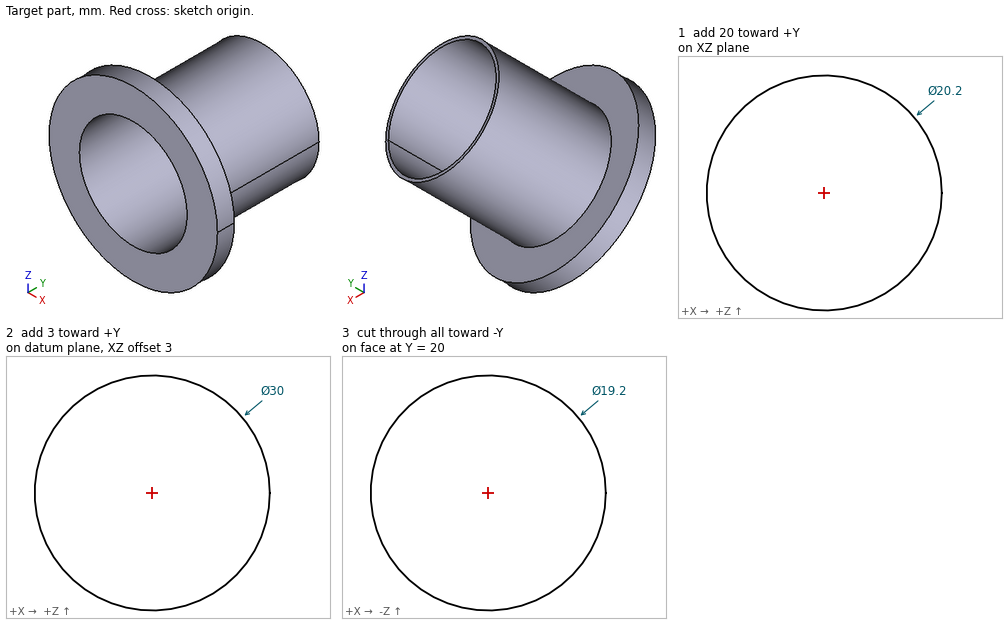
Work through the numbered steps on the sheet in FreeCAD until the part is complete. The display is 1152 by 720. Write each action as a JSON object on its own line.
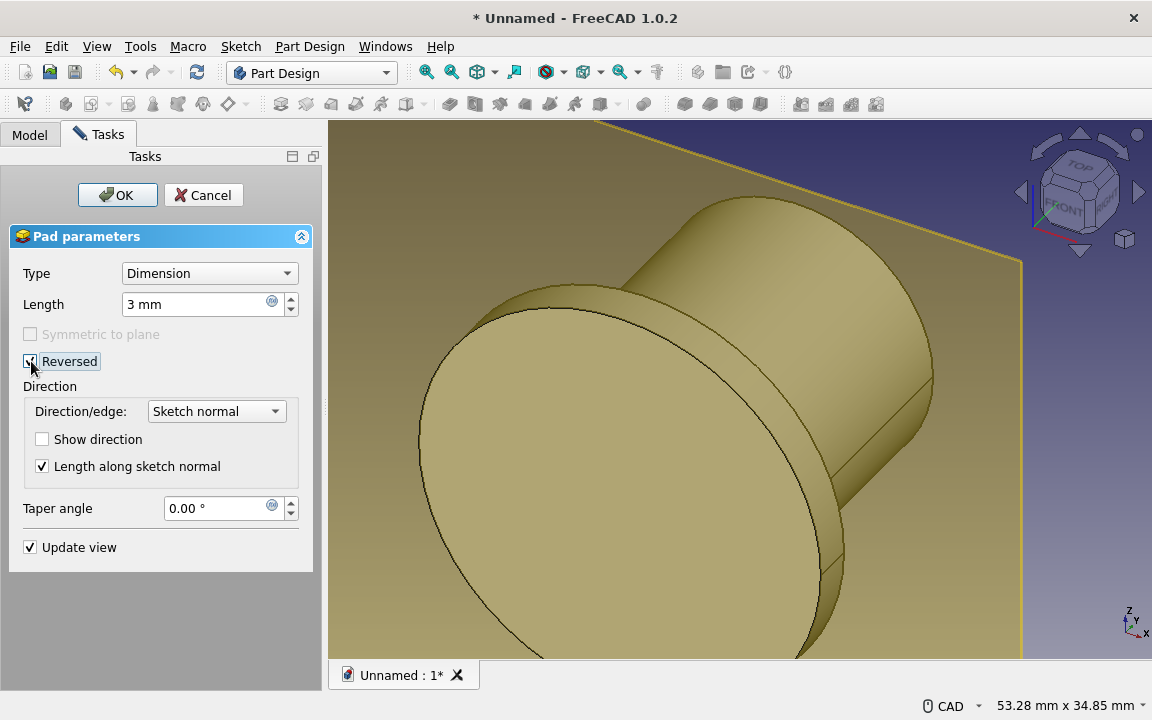
{"action": "left_click", "coordinate": [118, 195]}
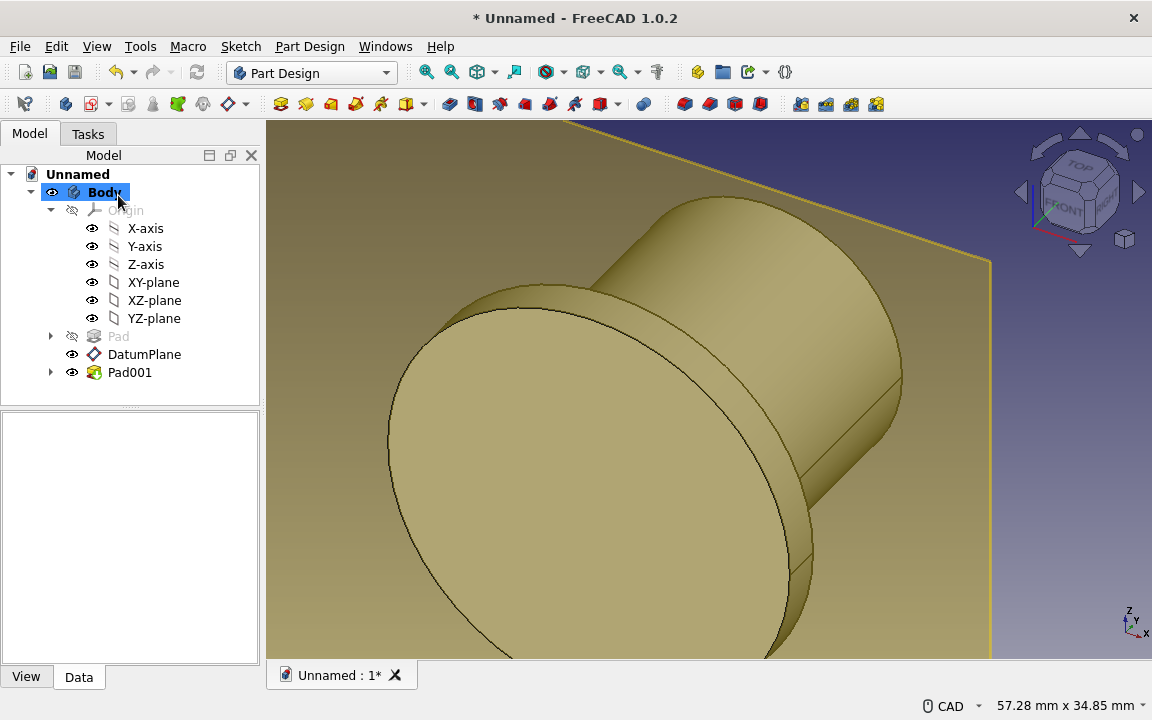
{"action": "left_click", "coordinate": [117, 354]}
{"action": "key", "text": "space"}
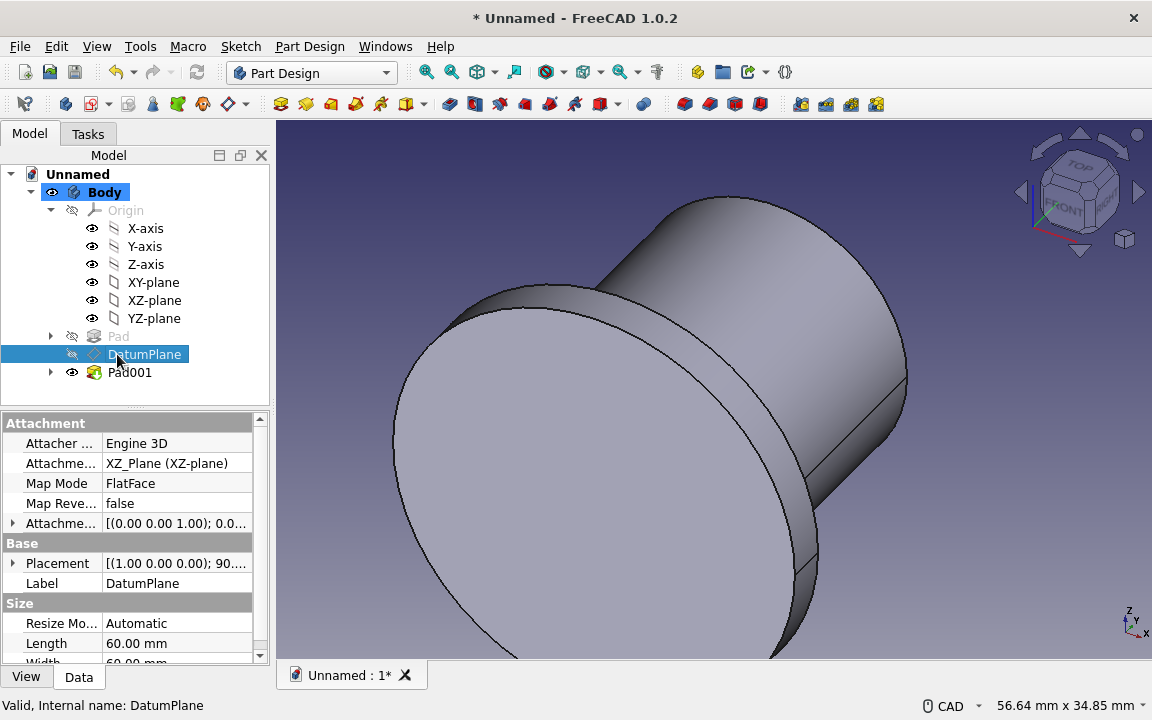
{"action": "key", "text": "v f"}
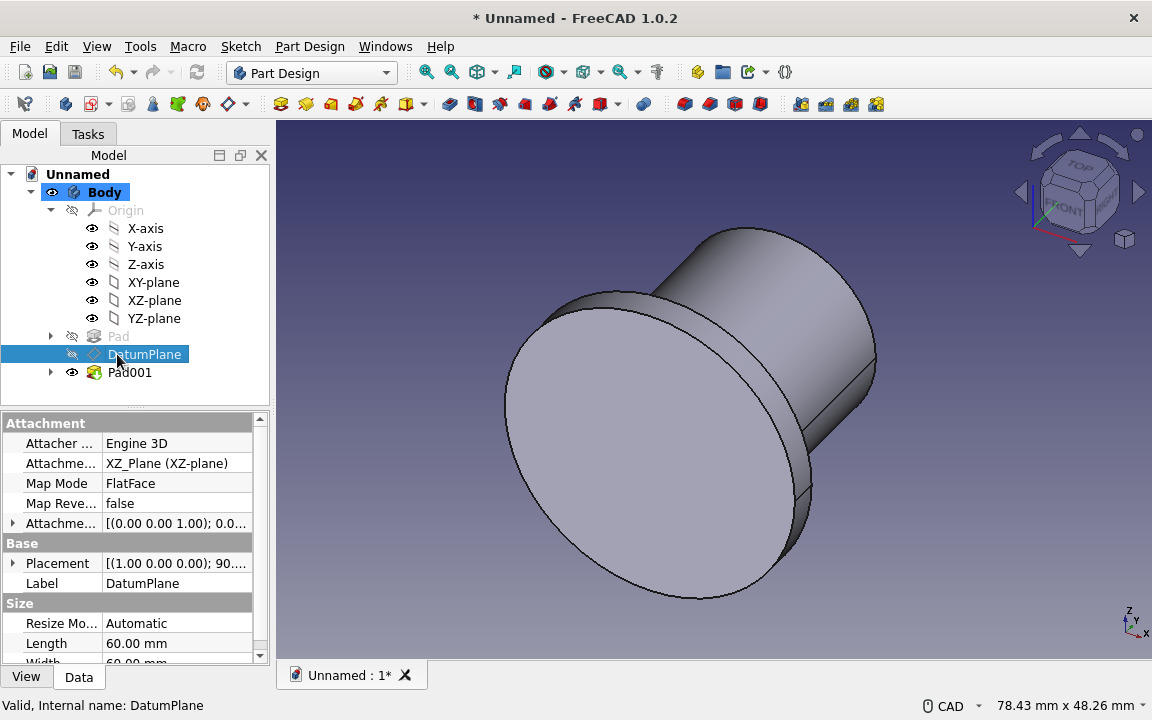
{"action": "key", "text": "4"}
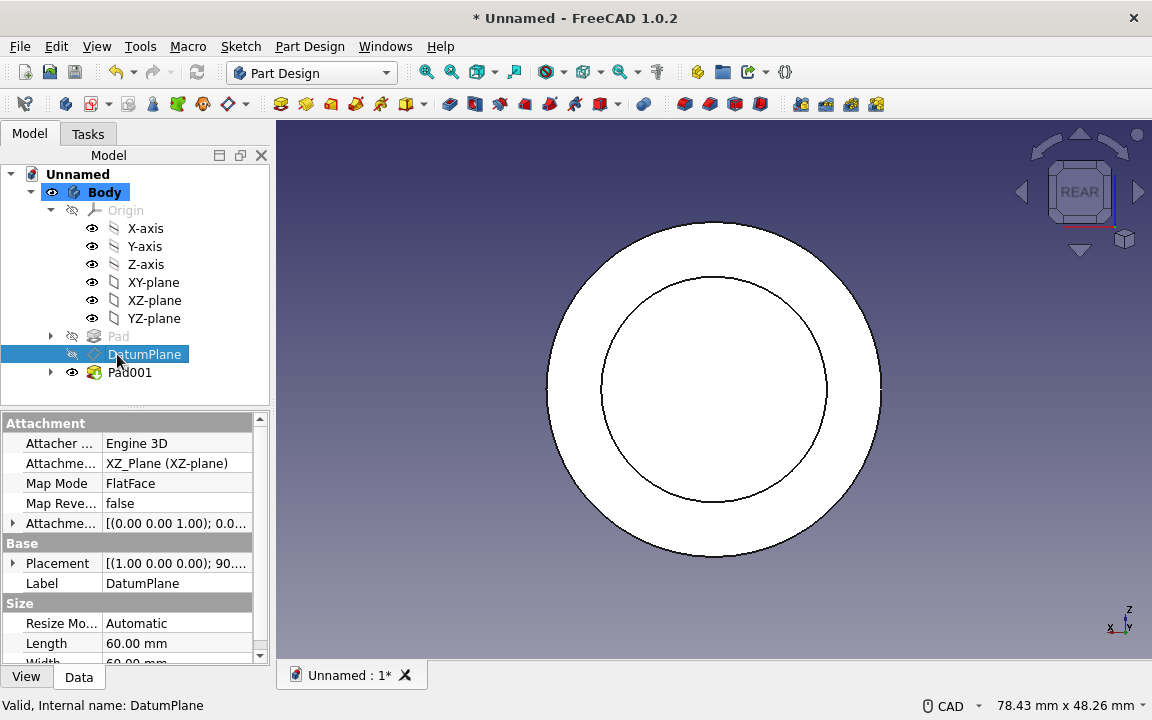
{"action": "left_click", "coordinate": [714, 389]}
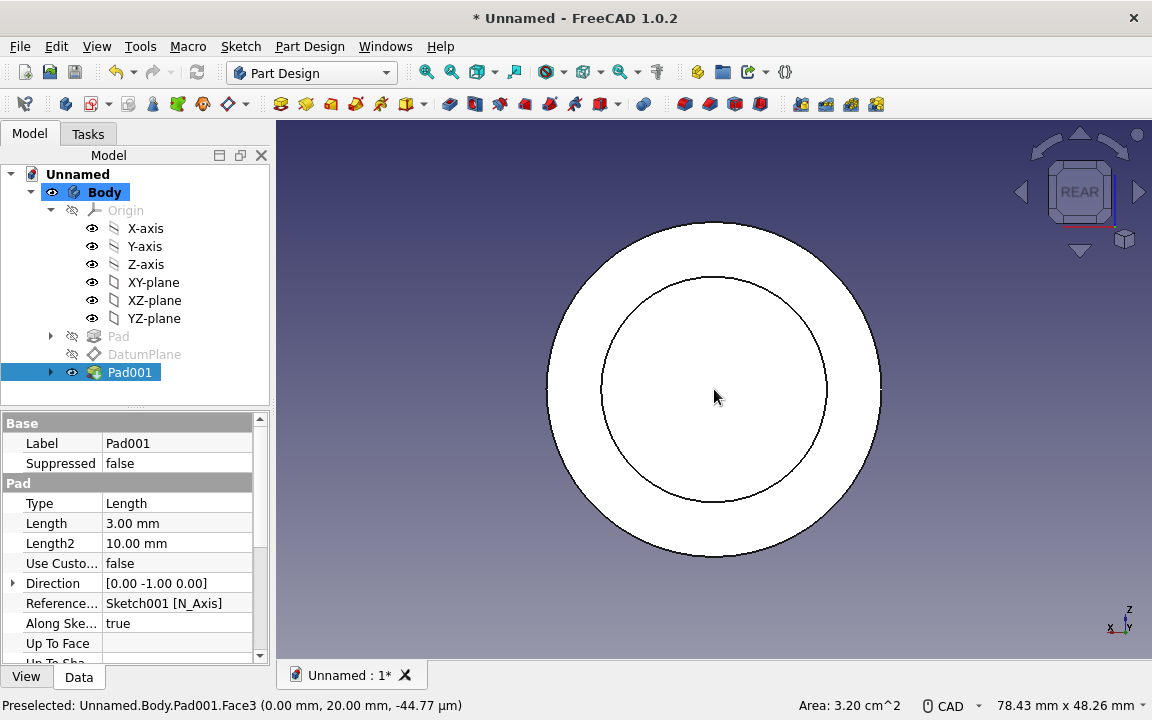
{"action": "left_click", "coordinate": [90, 104]}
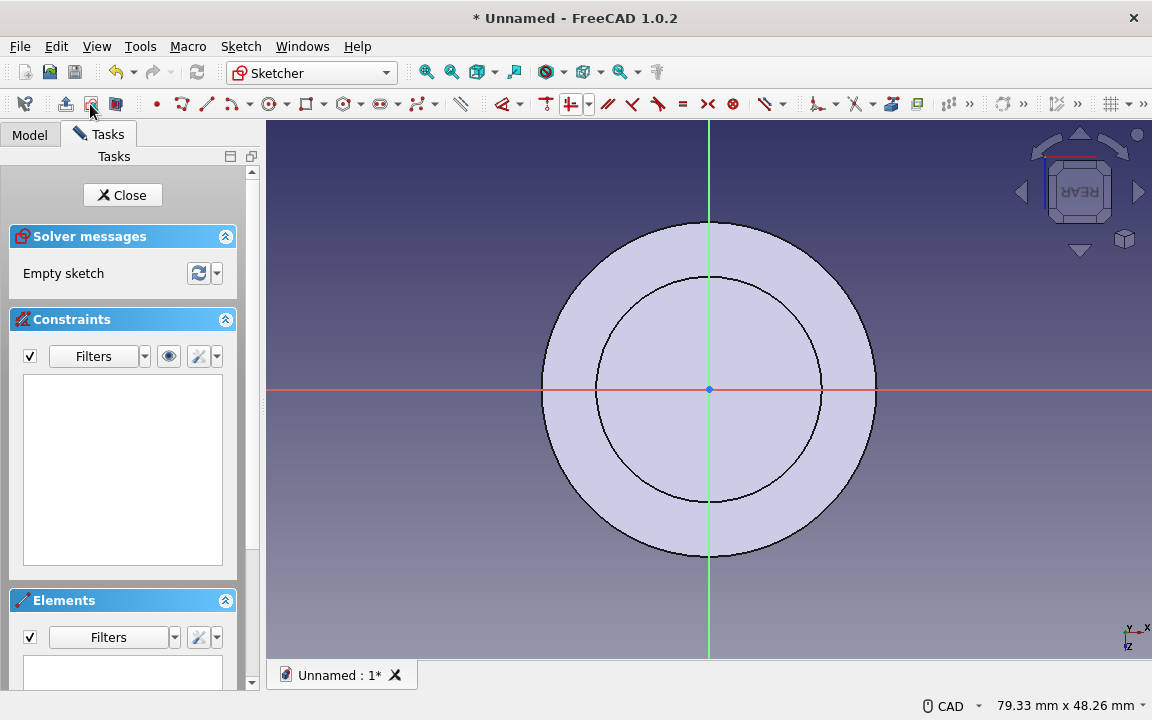
{"action": "scroll", "coordinate": [848, 390], "scroll_direction": "up", "scroll_amount": 2}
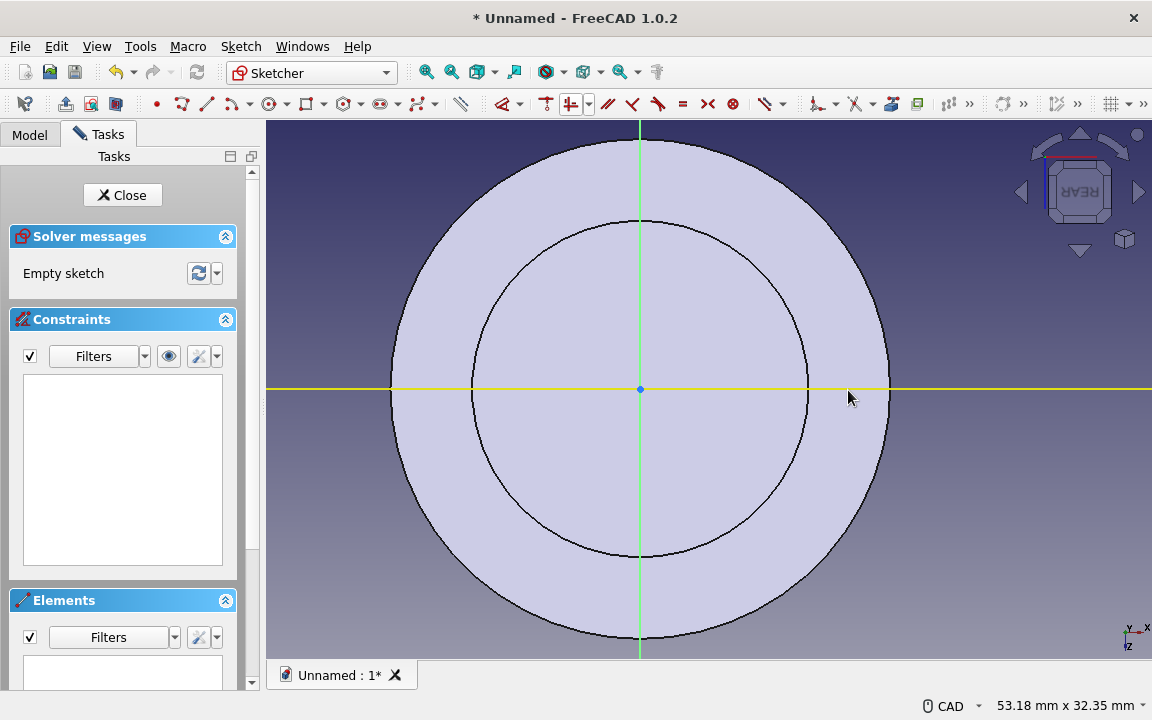
{"action": "key", "text": "g c"}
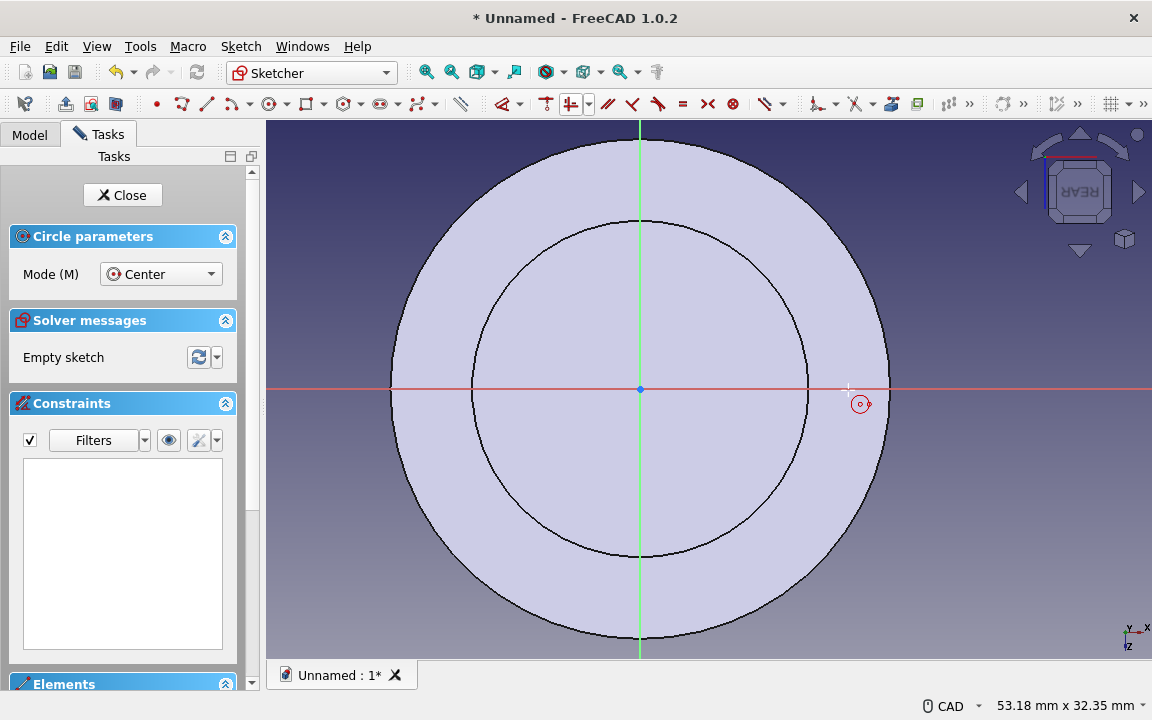
{"action": "left_click", "coordinate": [640, 389]}
{"action": "left_click", "coordinate": [753, 276]}
{"action": "key", "text": "Escape"}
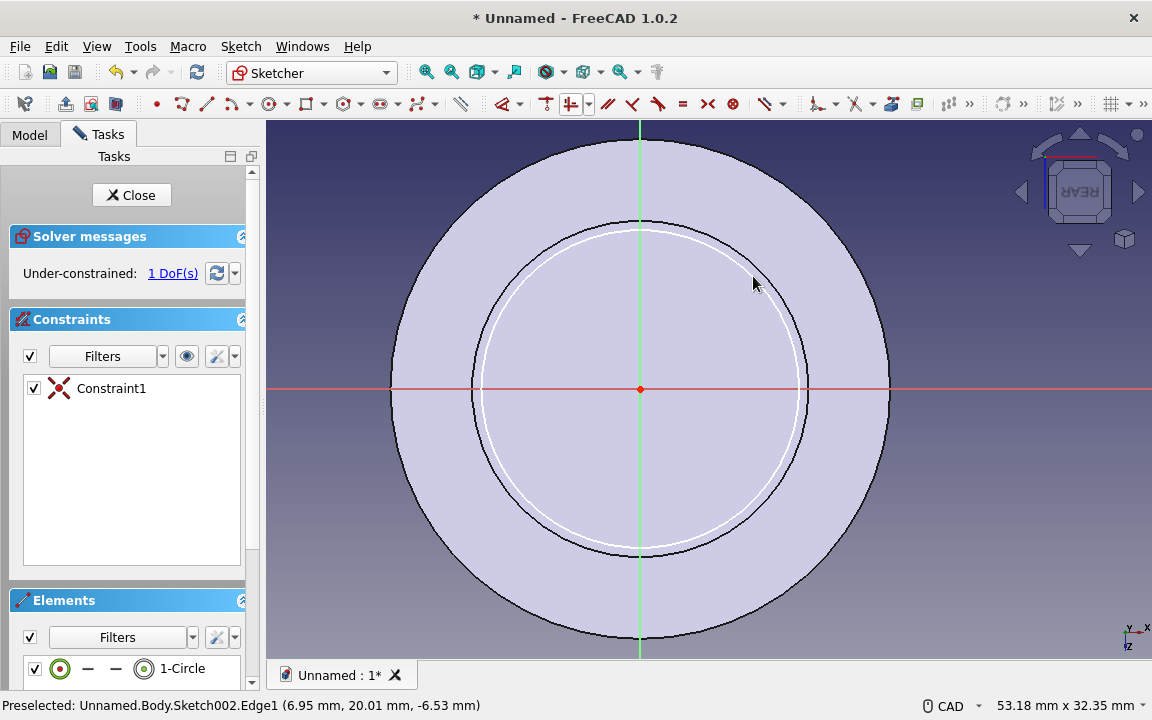
{"action": "left_click", "coordinate": [502, 104]}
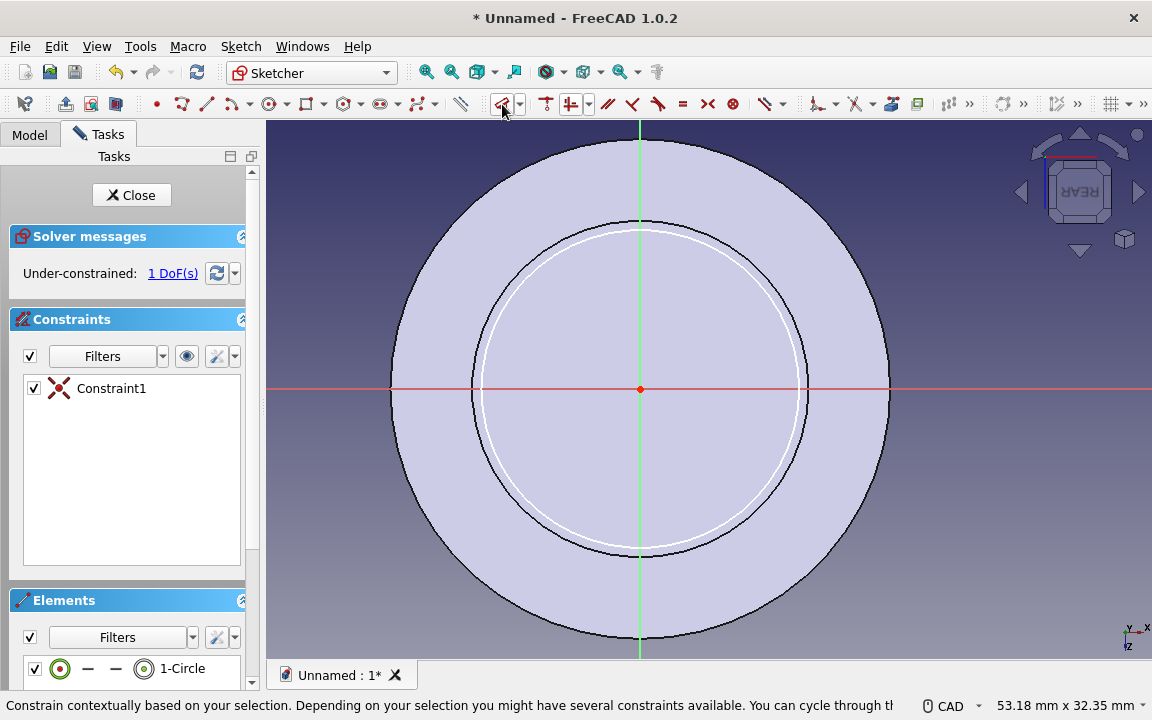
{"action": "left_click", "coordinate": [752, 276]}
{"action": "left_click", "coordinate": [774, 253]}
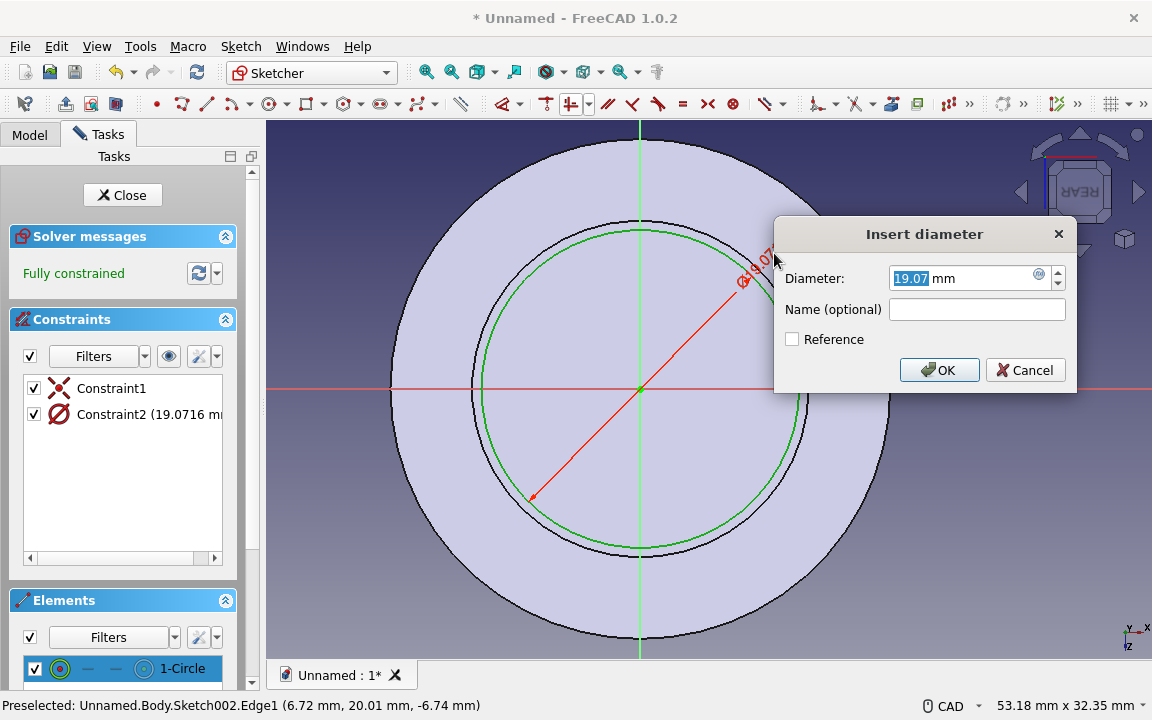
{"action": "type", "text": "19.2"}
{"action": "key", "text": "Return"}
{"action": "key", "text": "Escape"}